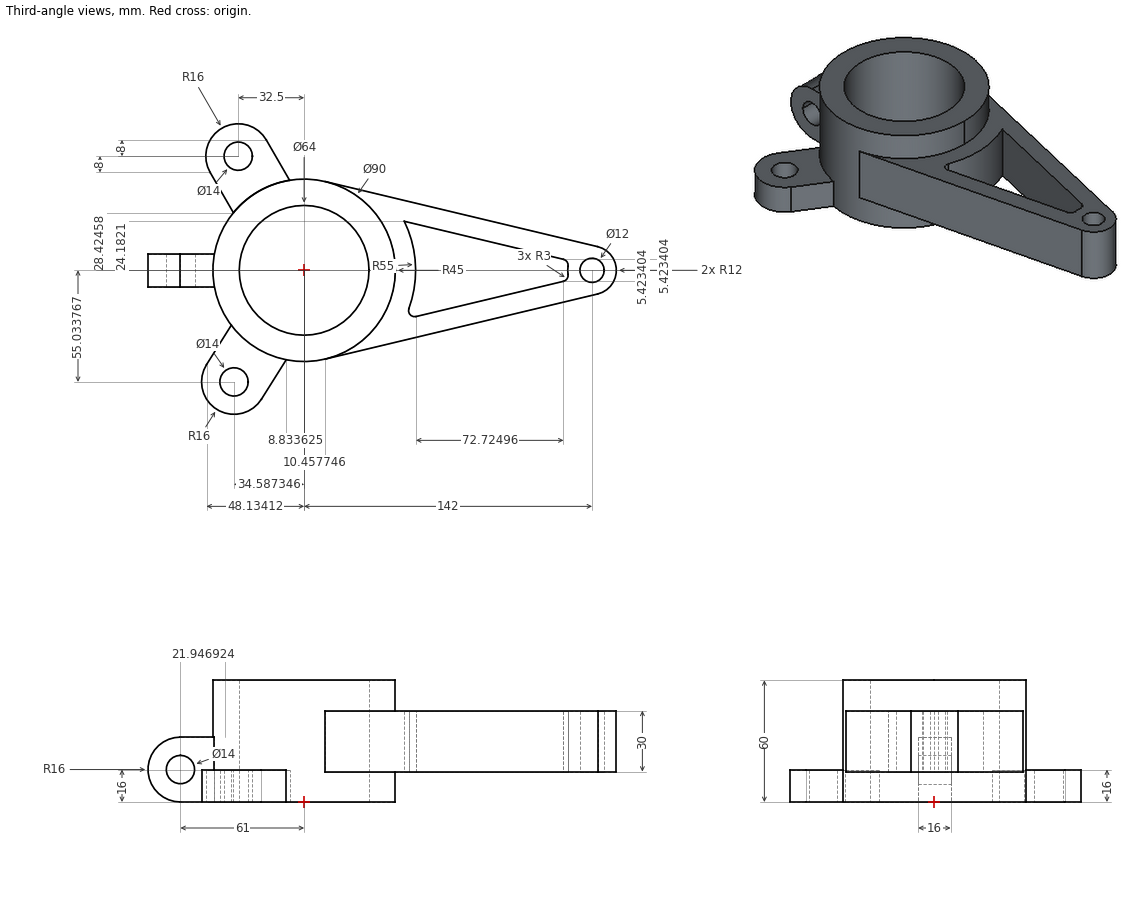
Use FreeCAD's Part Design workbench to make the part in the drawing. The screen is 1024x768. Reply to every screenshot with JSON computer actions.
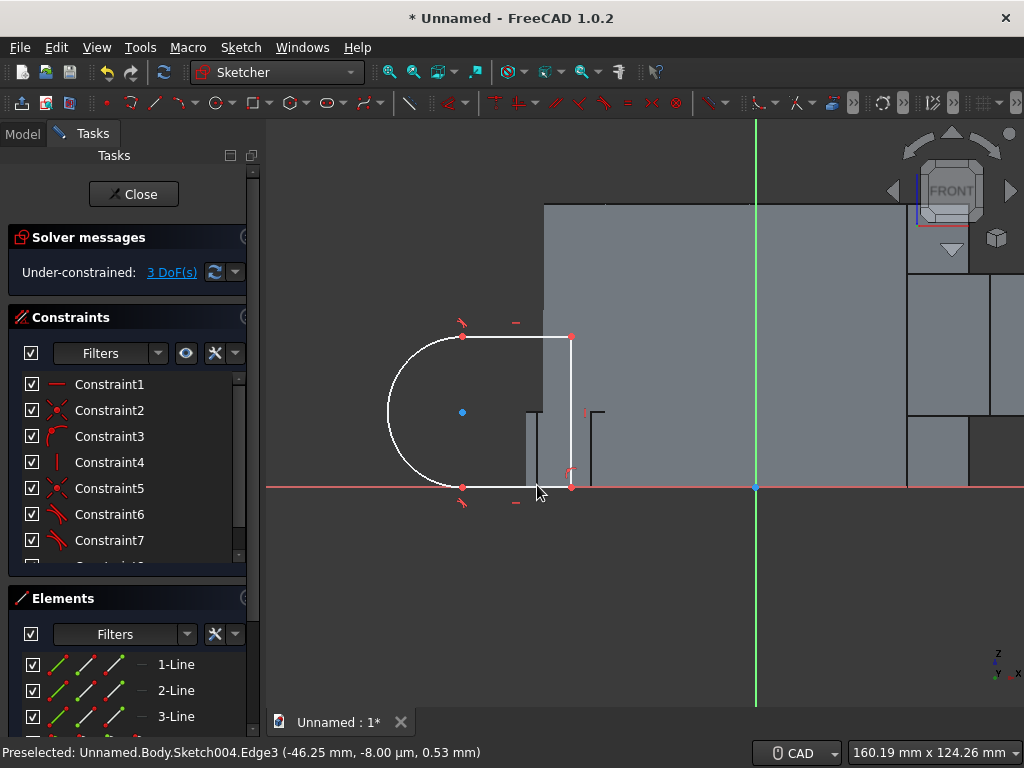
{"action": "key", "text": "d"}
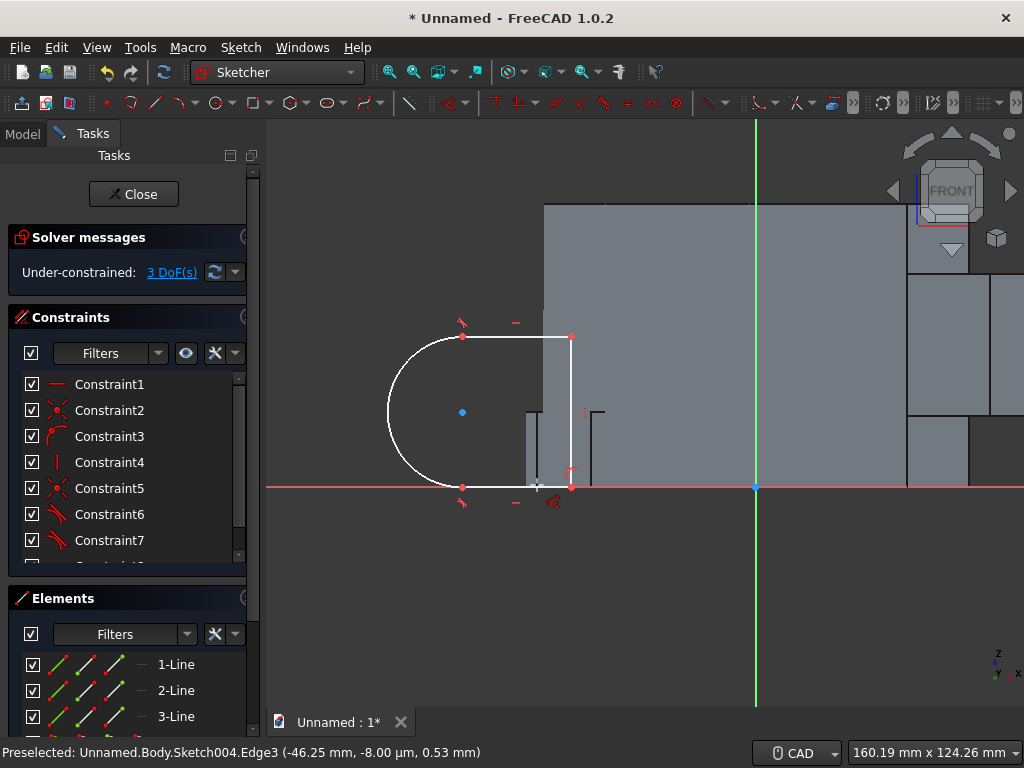
{"action": "left_click", "coordinate": [402, 368]}
{"action": "left_click", "coordinate": [376, 349]}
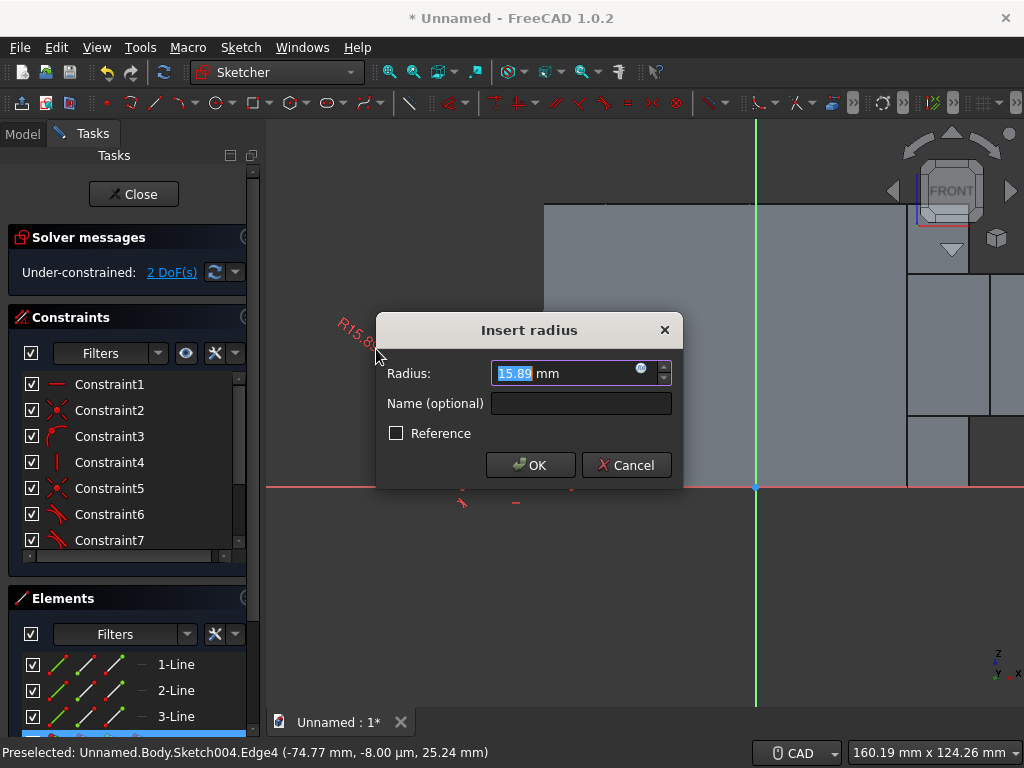
{"action": "type", "text": "16"}
{"action": "key", "text": "Return"}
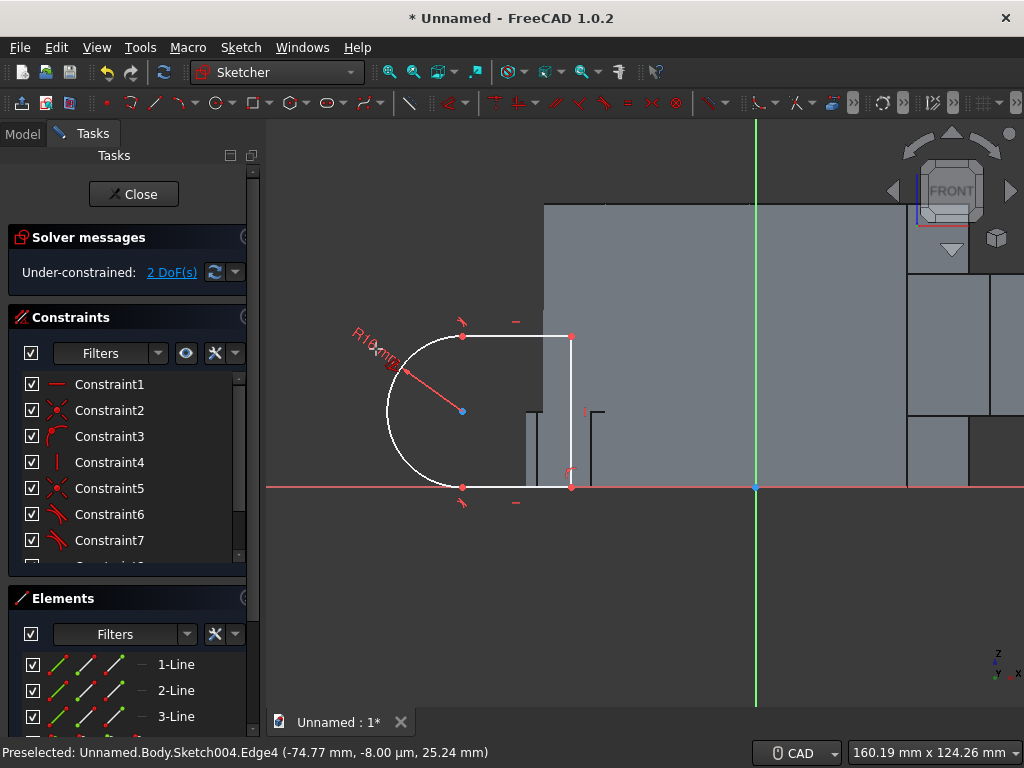
{"action": "left_click", "coordinate": [463, 336]}
{"action": "left_click", "coordinate": [609, 521]}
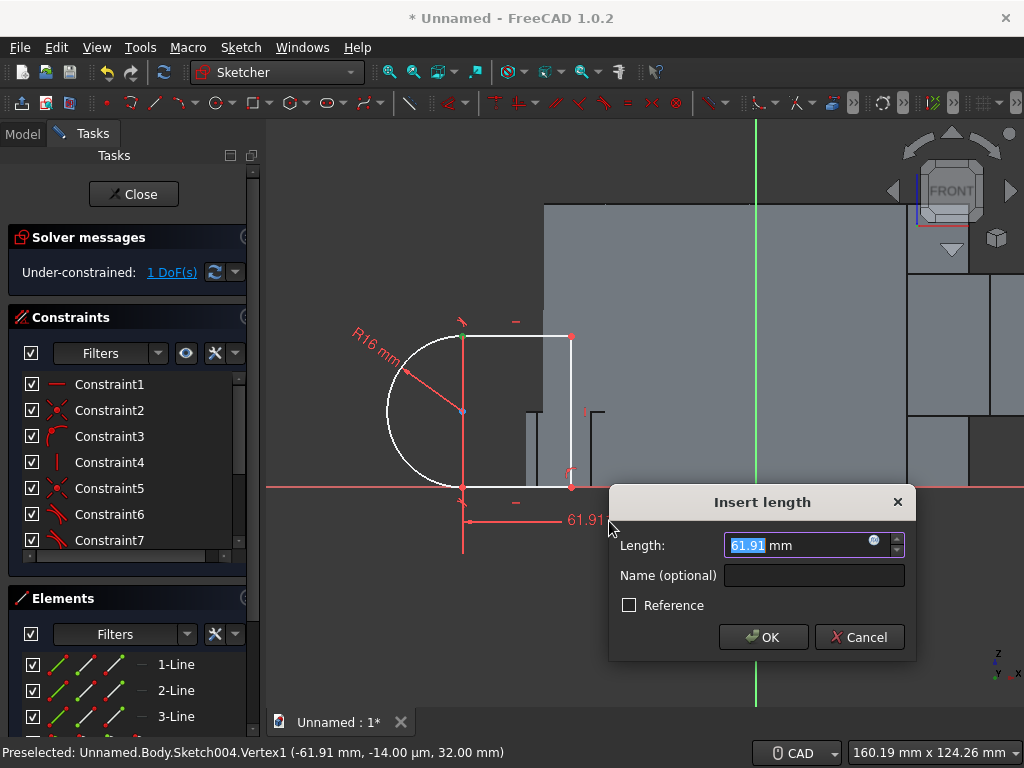
{"action": "type", "text": "61"}
{"action": "key", "text": "Return"}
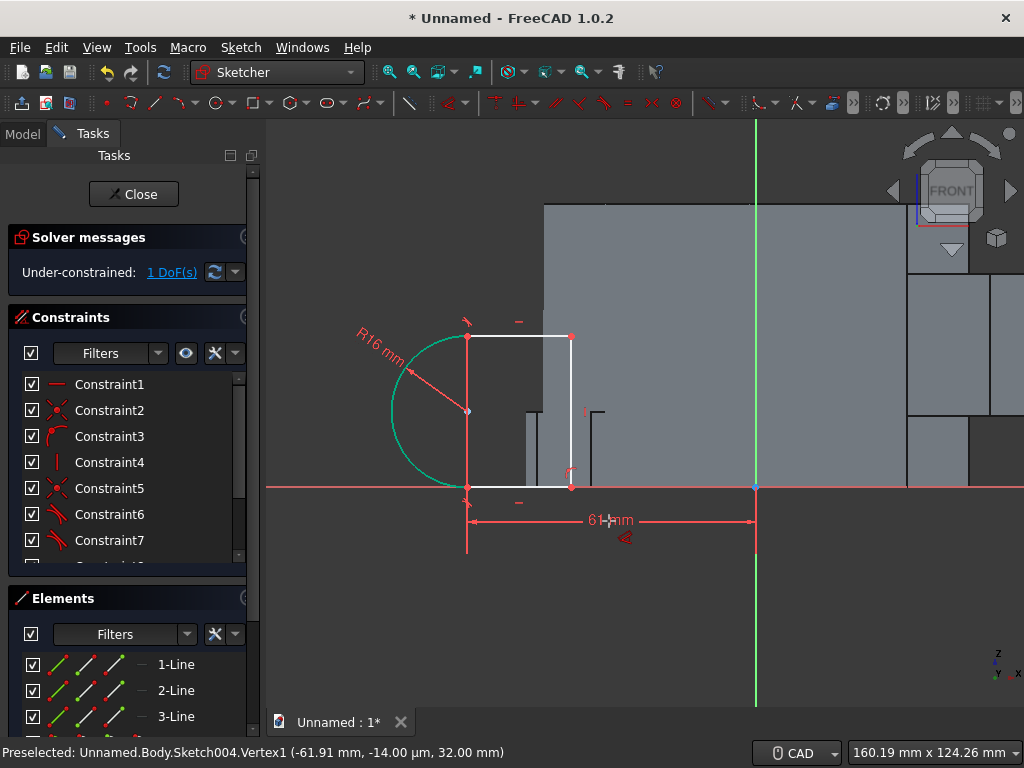
{"action": "left_click", "coordinate": [498, 336]}
{"action": "left_click", "coordinate": [519, 302]}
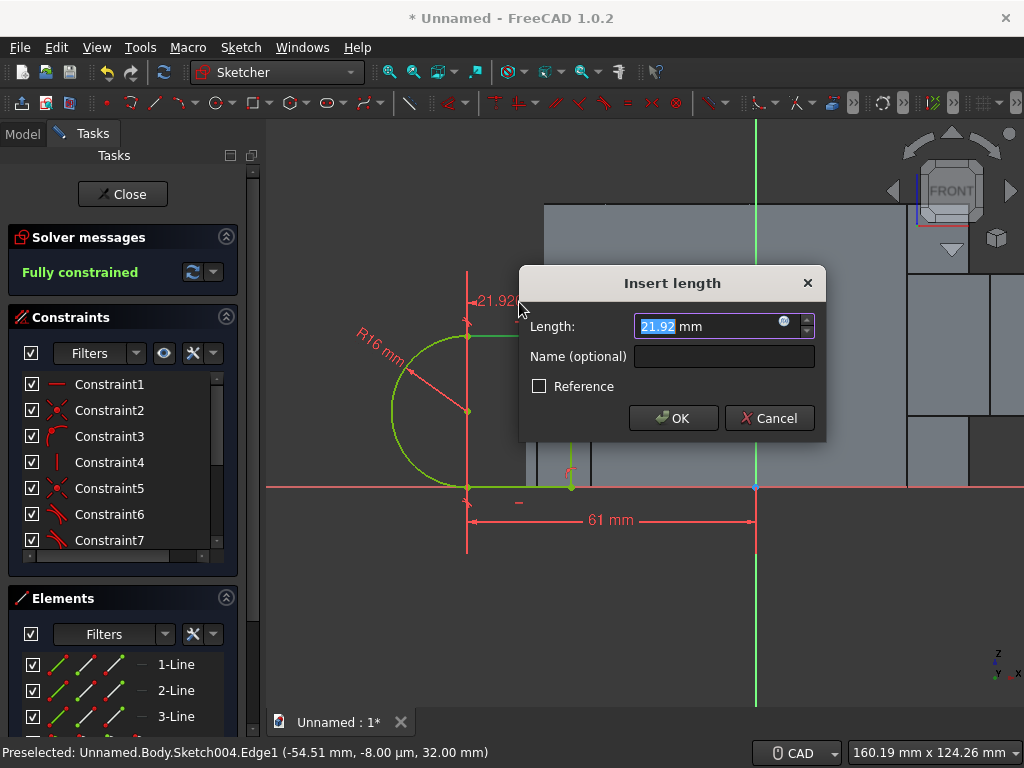
{"action": "type", "text": "21.946924"}
{"action": "key", "text": "Return"}
{"action": "key", "text": "Escape"}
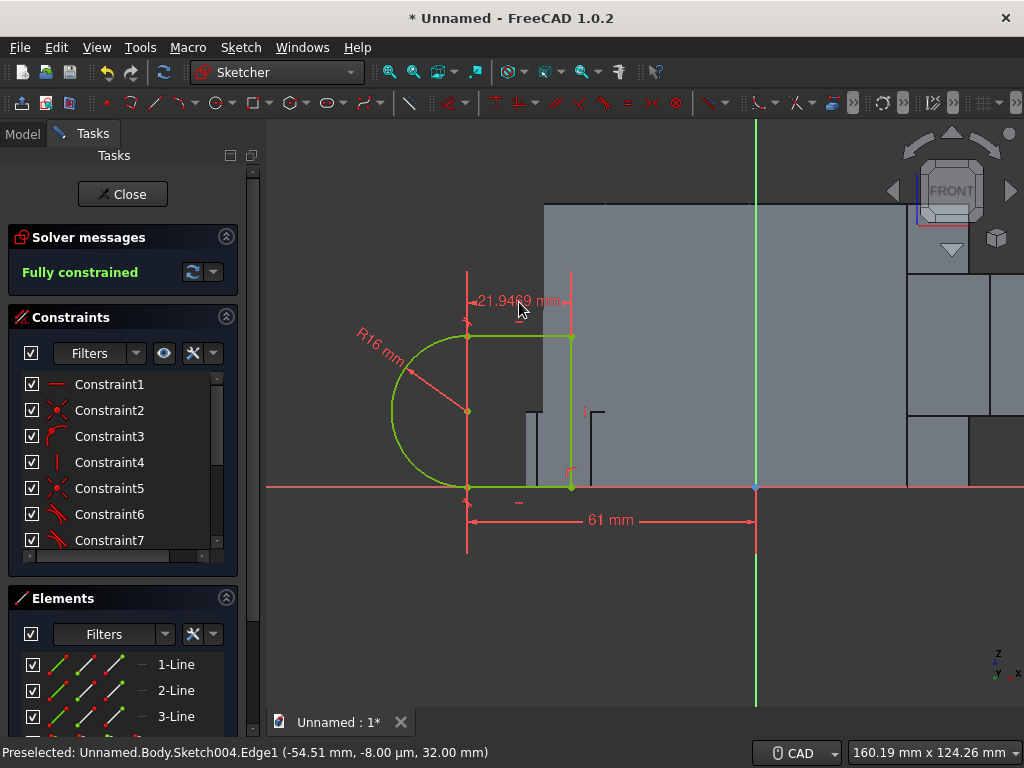
{"action": "left_click", "coordinate": [123, 194]}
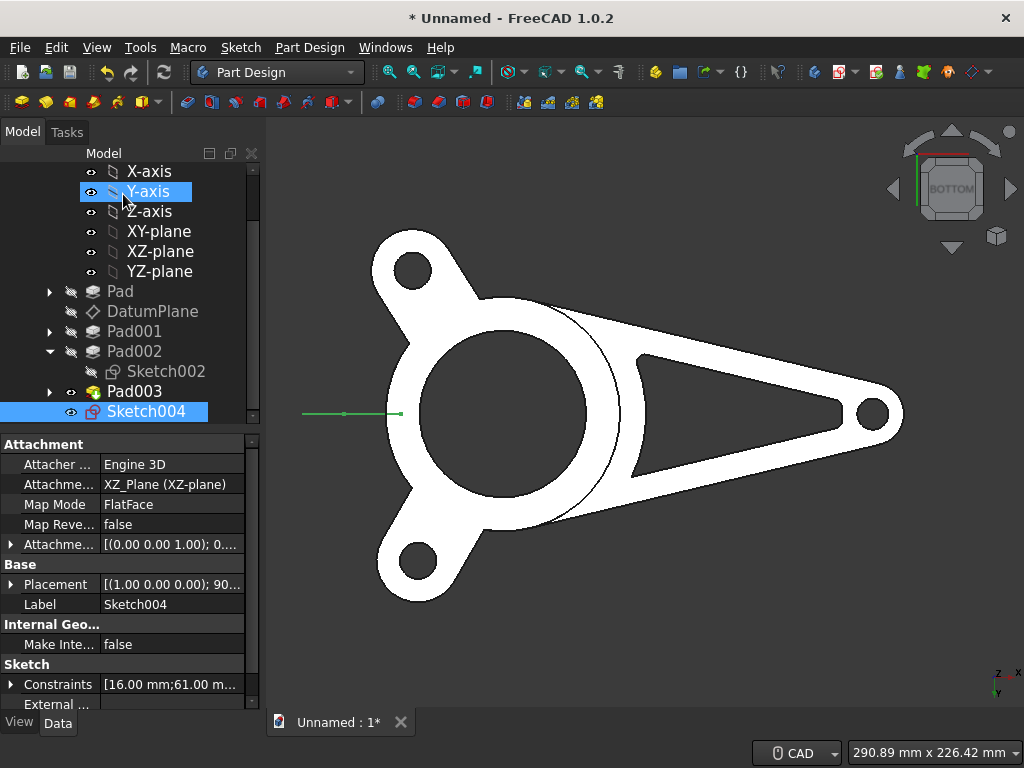
{"action": "left_click", "coordinate": [22, 102]}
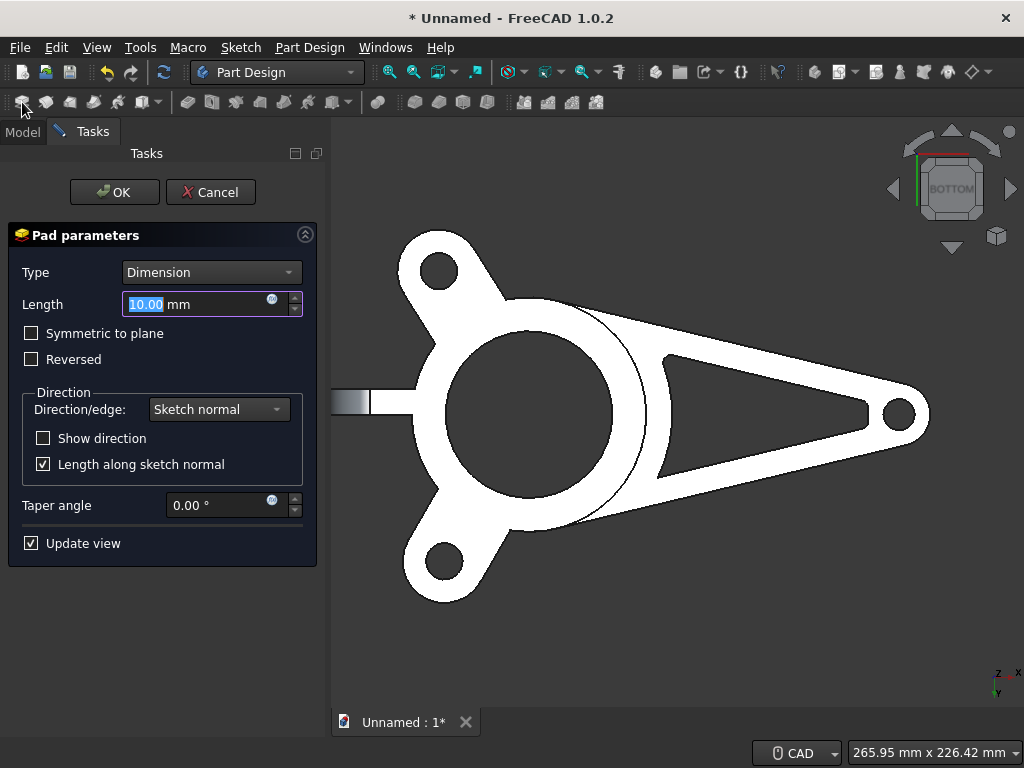
{"action": "type", "text": "16"}
{"action": "key", "text": "Tab"}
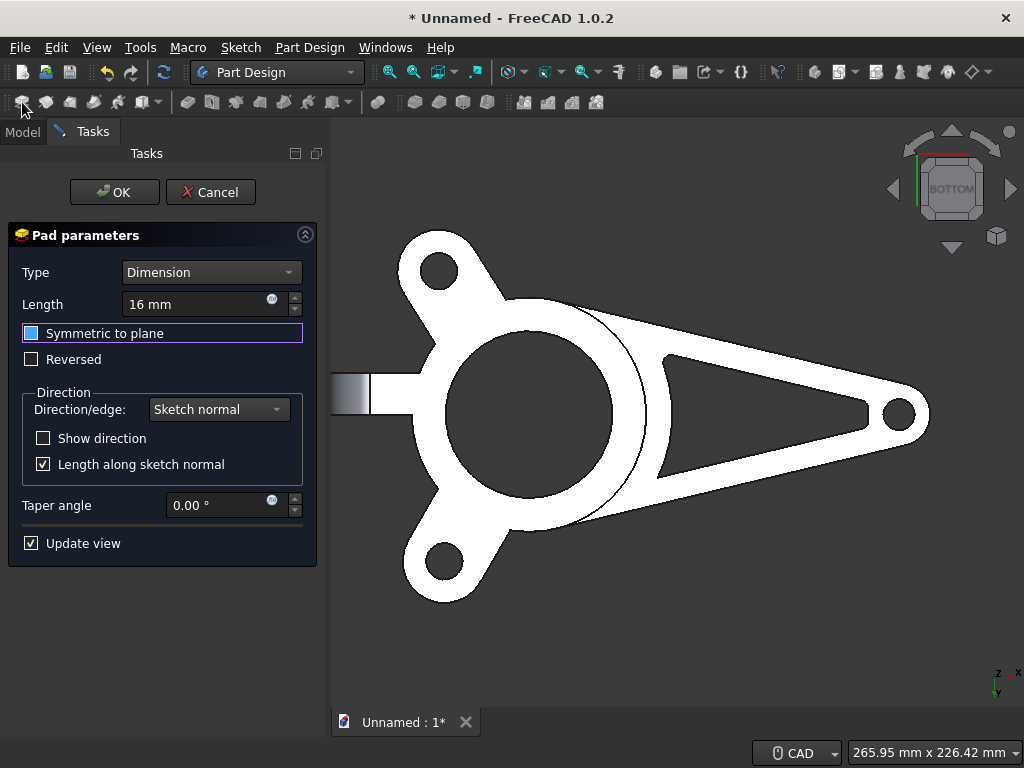
{"action": "left_click", "coordinate": [30, 333]}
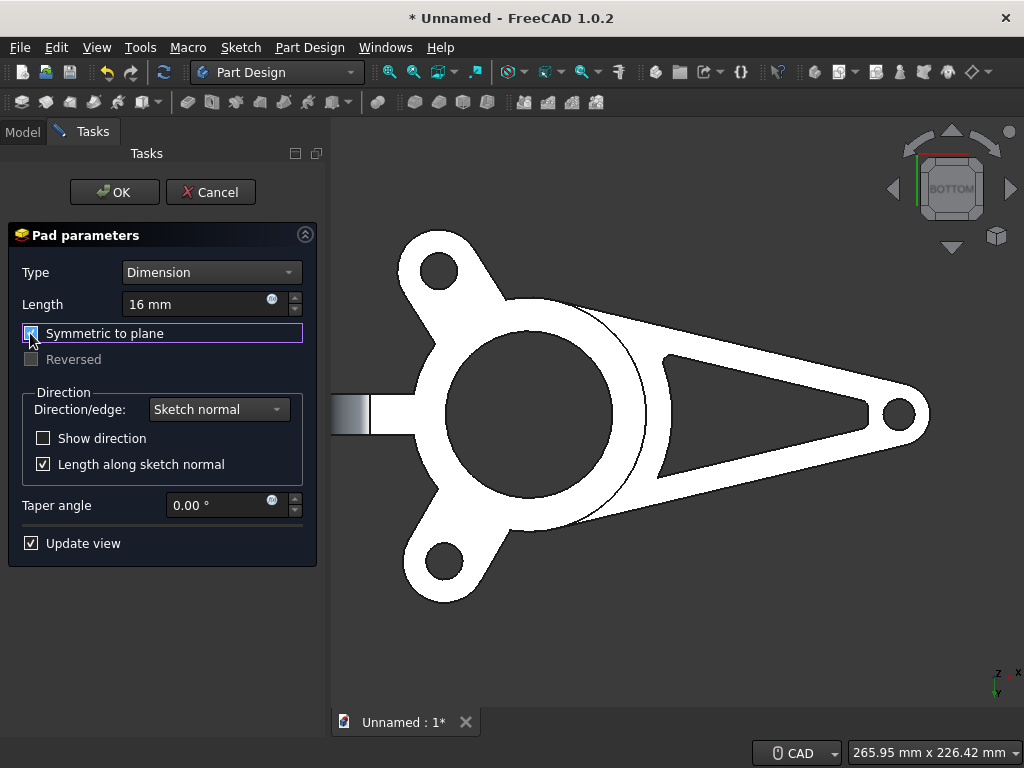
{"action": "left_click", "coordinate": [115, 192]}